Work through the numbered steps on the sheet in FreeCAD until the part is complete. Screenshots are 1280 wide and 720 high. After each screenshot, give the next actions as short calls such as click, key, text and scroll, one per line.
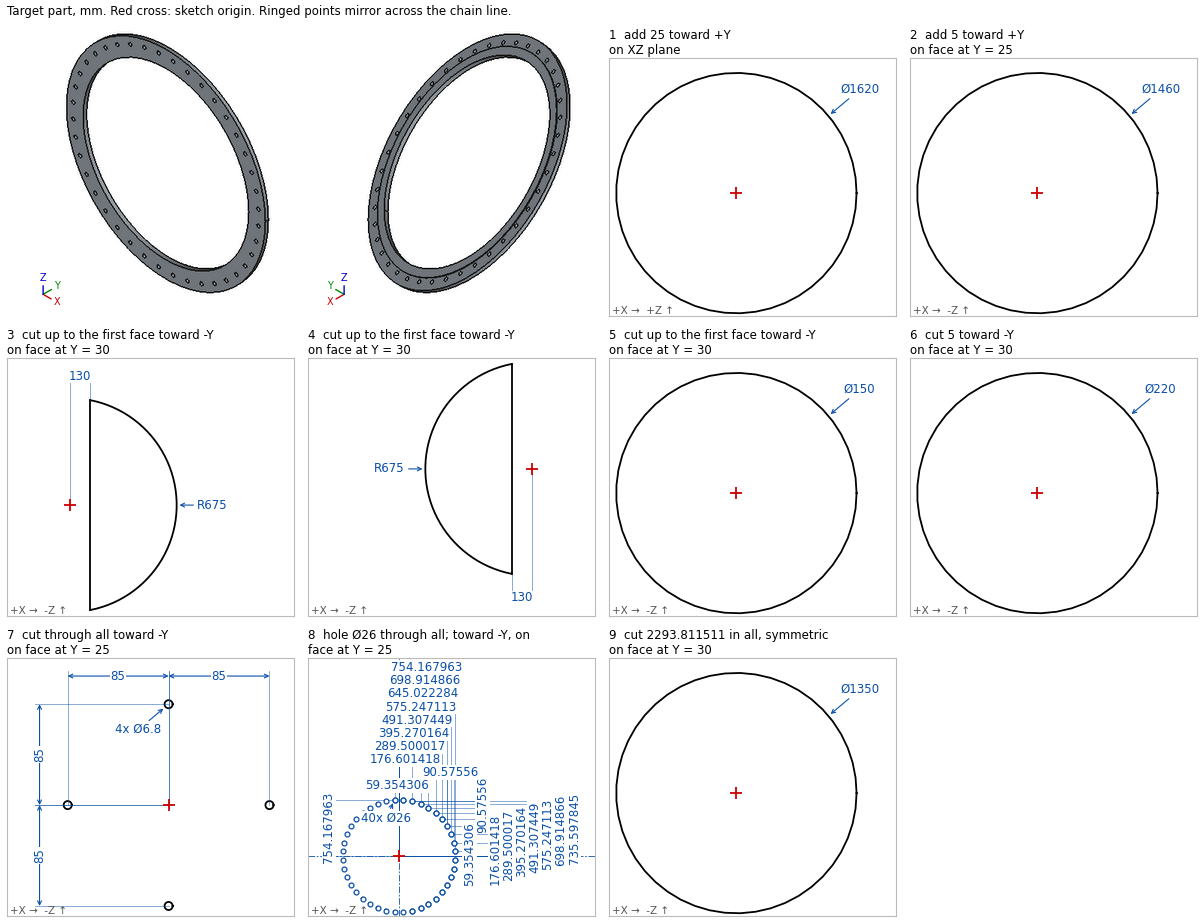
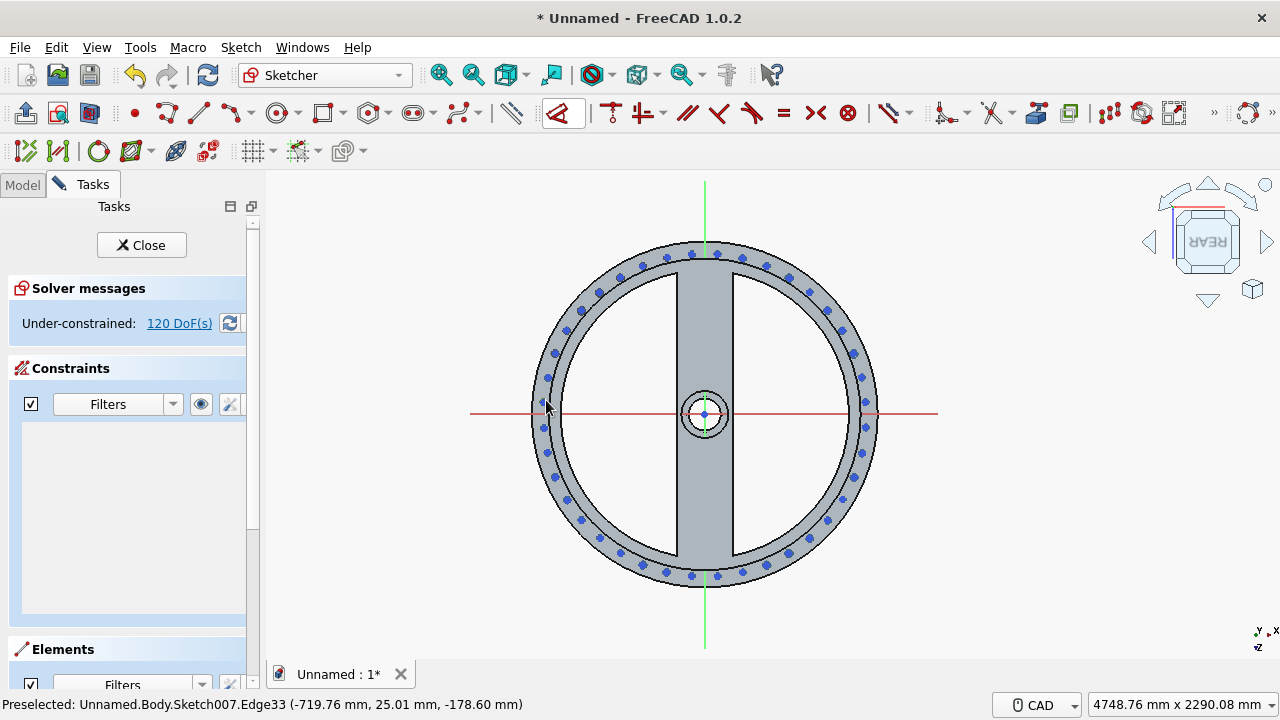
scroll(558, 351, up, 7)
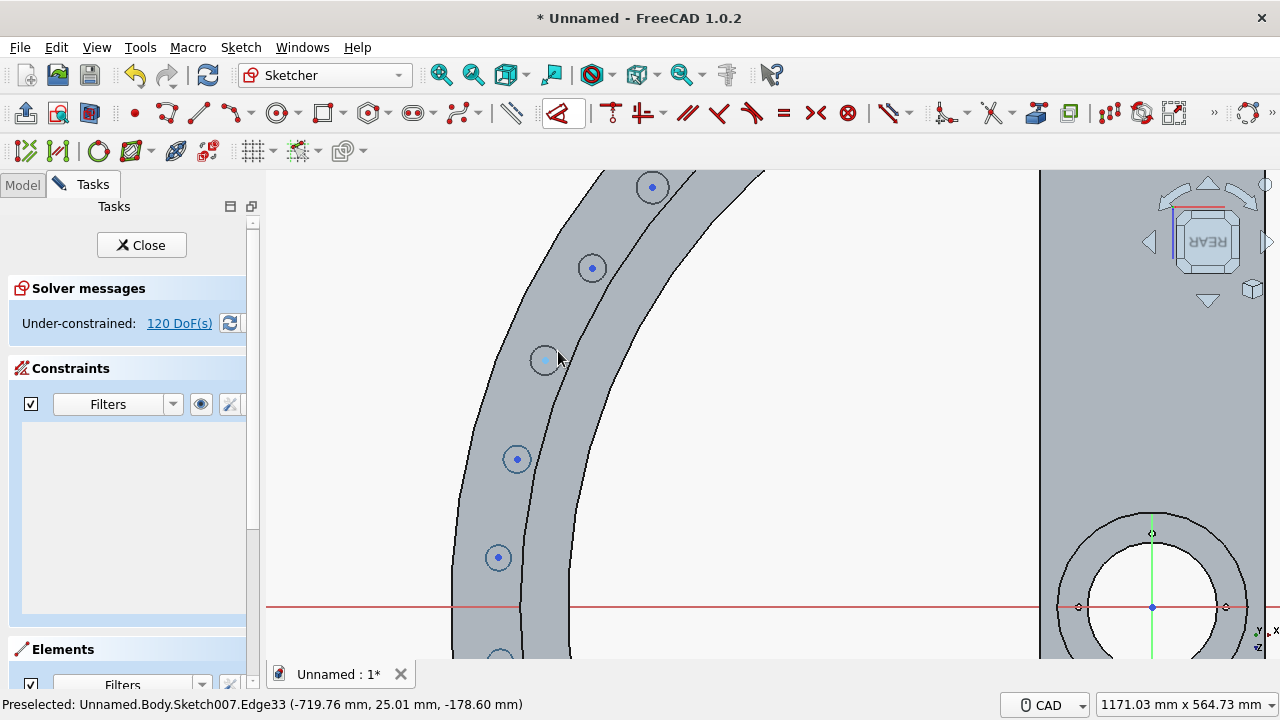
click(555, 350)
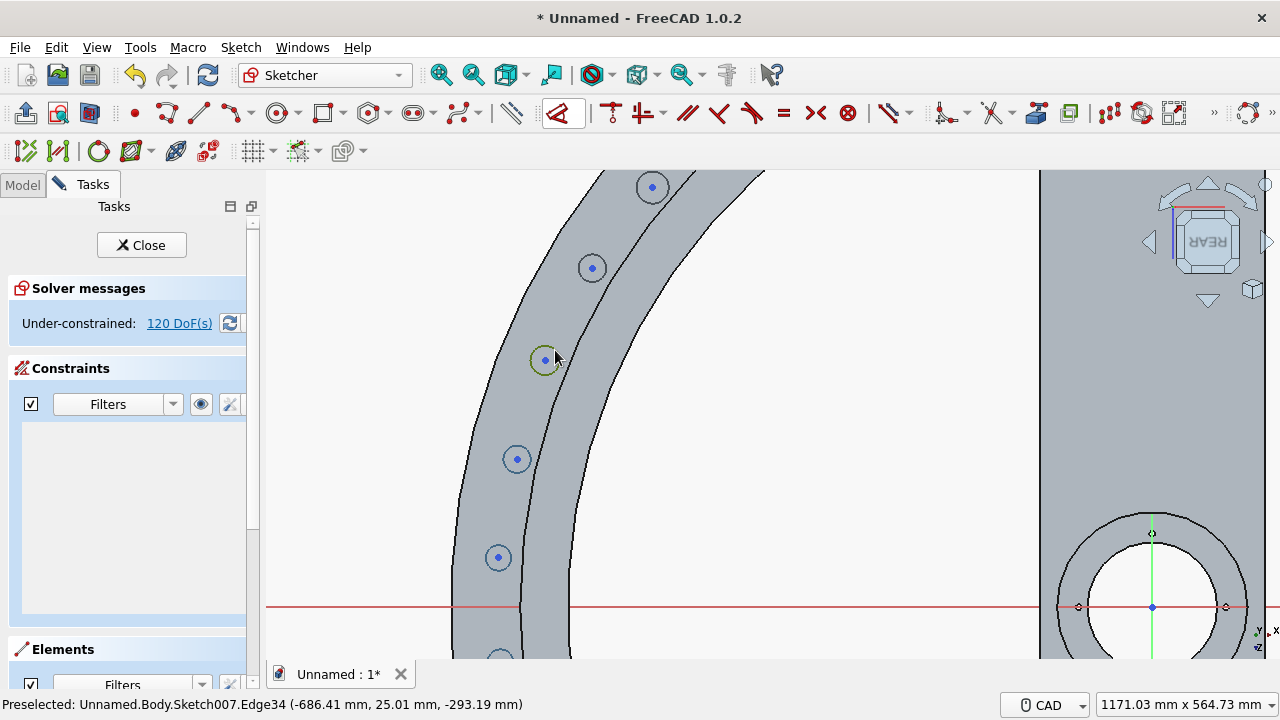
click(602, 258)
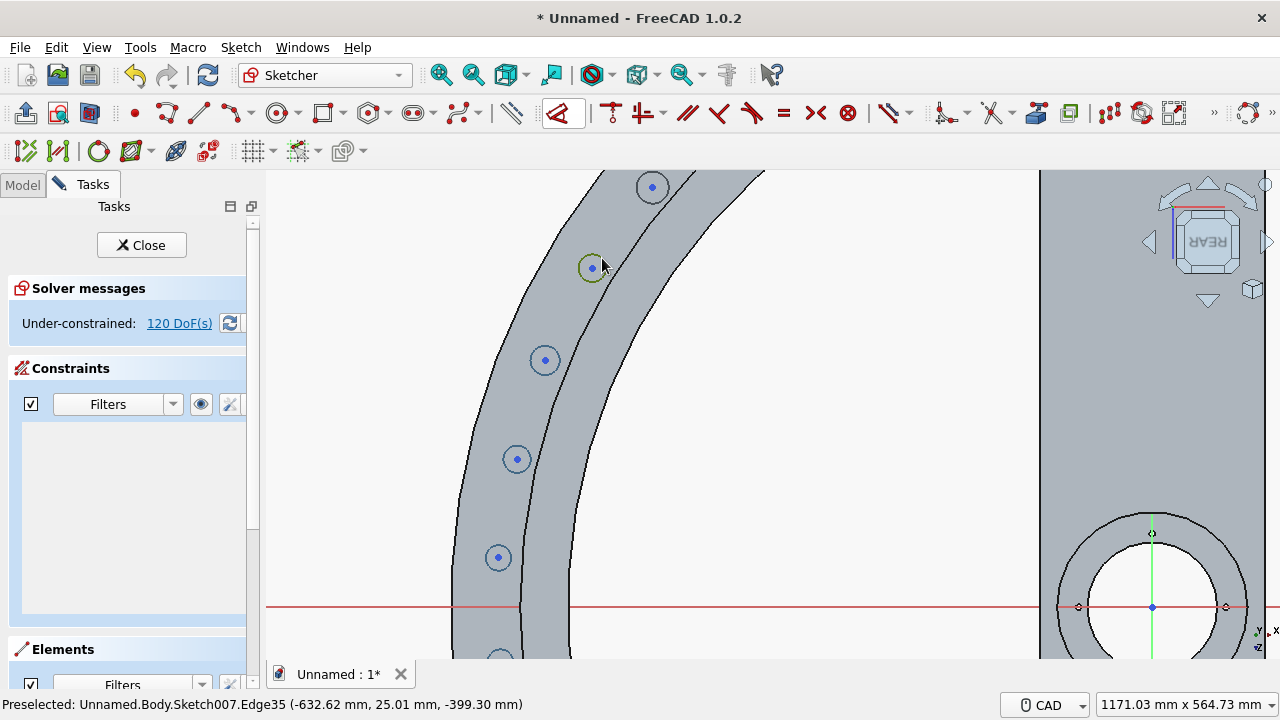
click(641, 199)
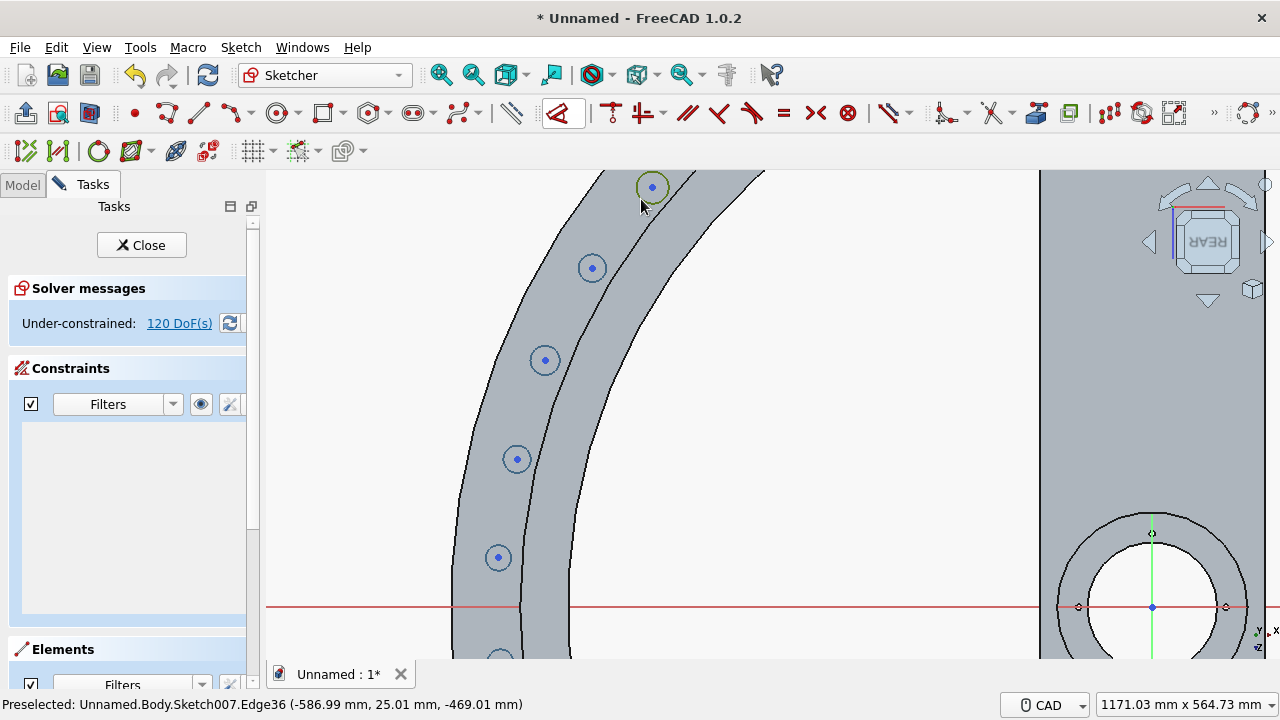
scroll(558, 351, down, 7)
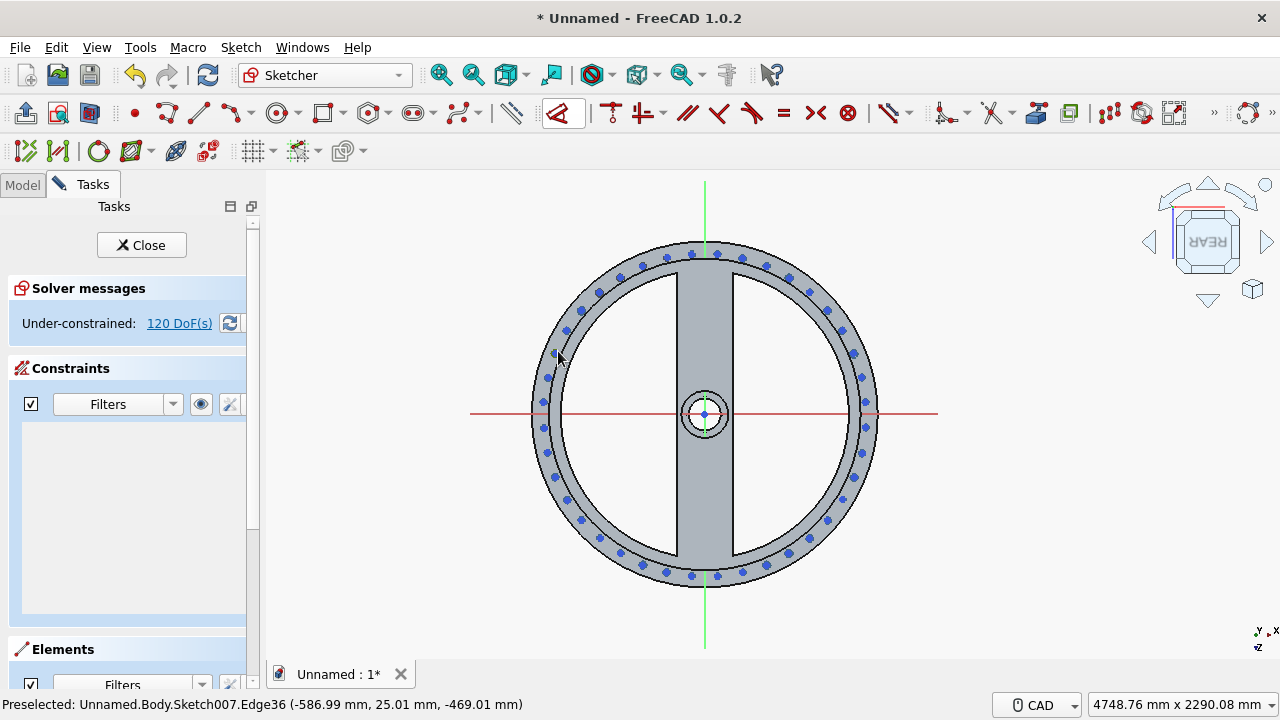
scroll(602, 290, up, 7)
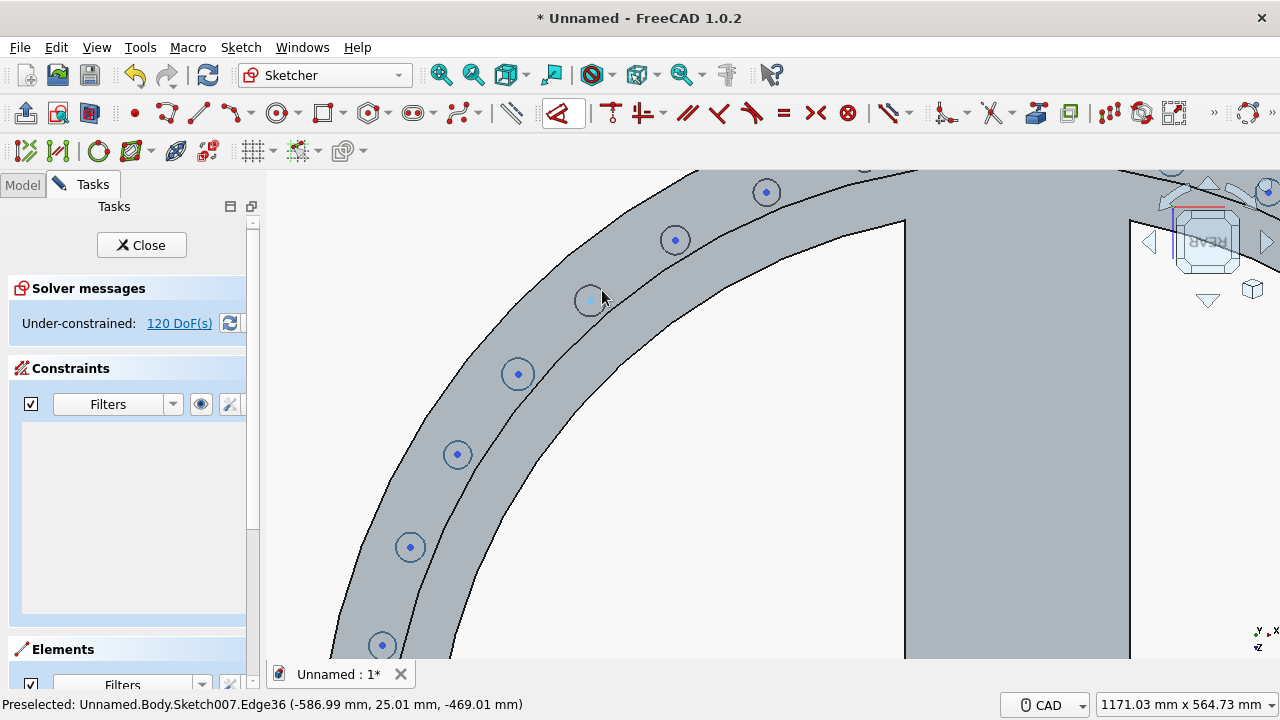
click(601, 290)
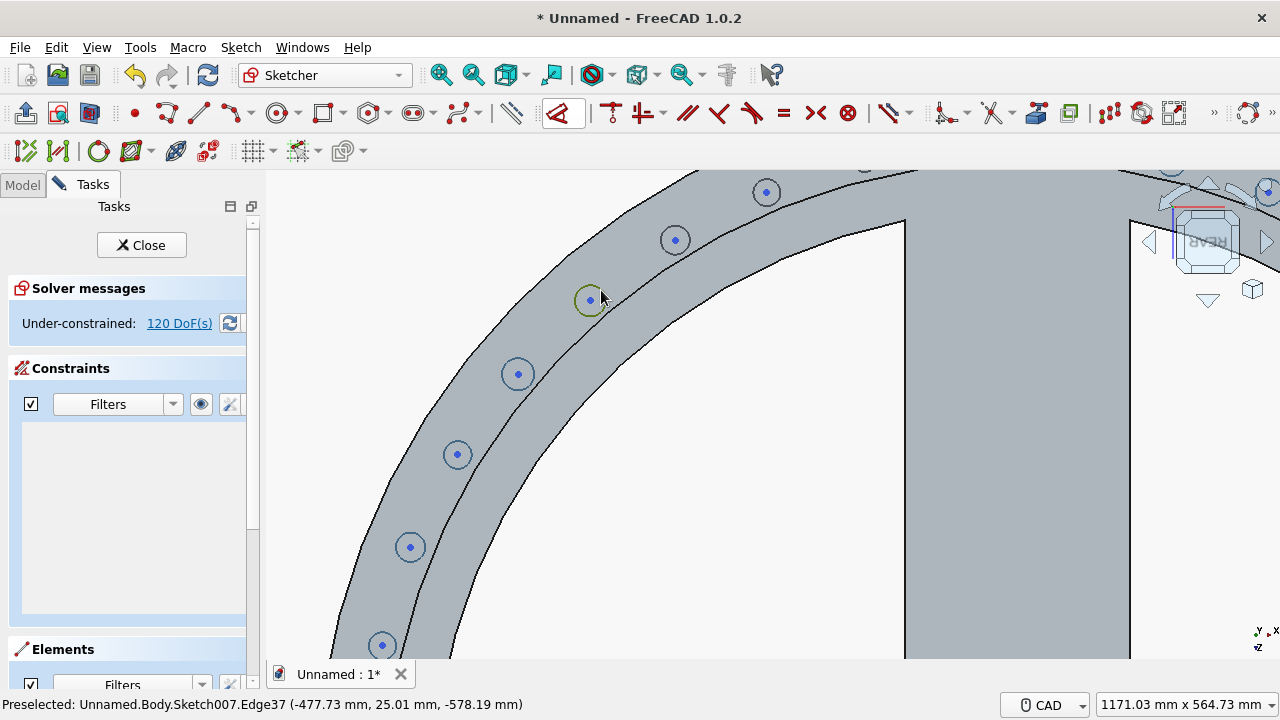
click(686, 230)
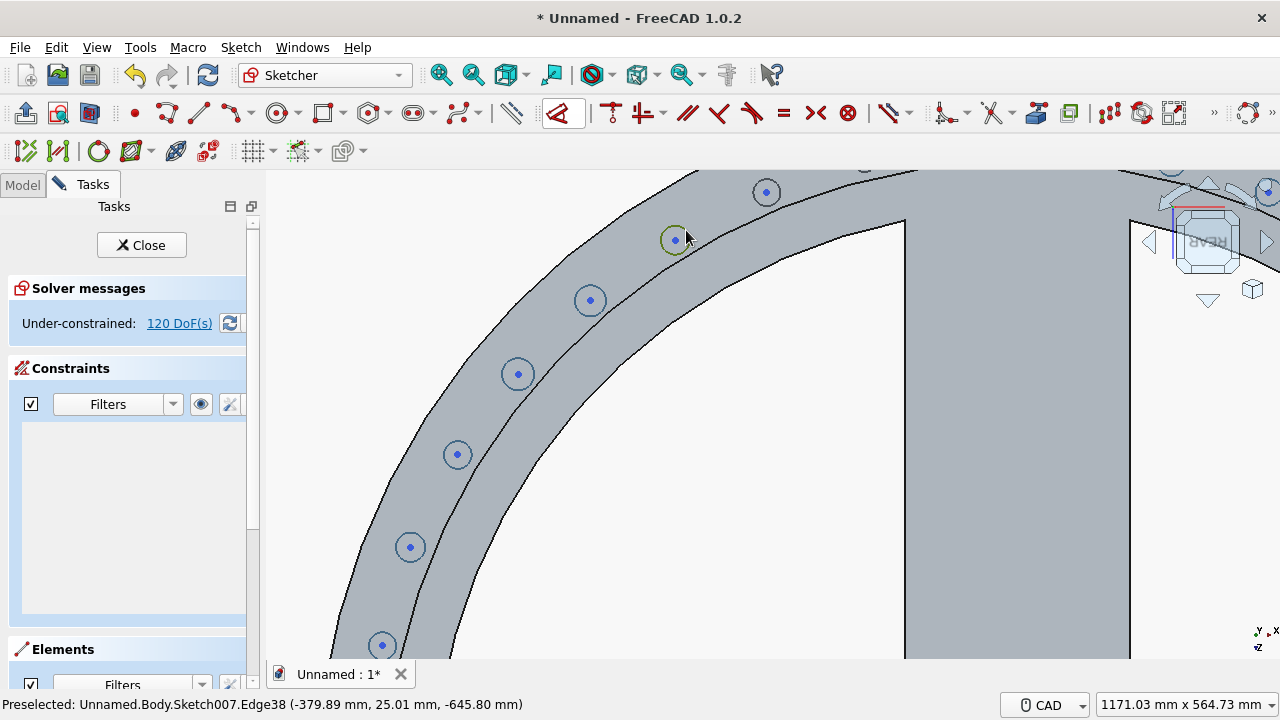
click(757, 202)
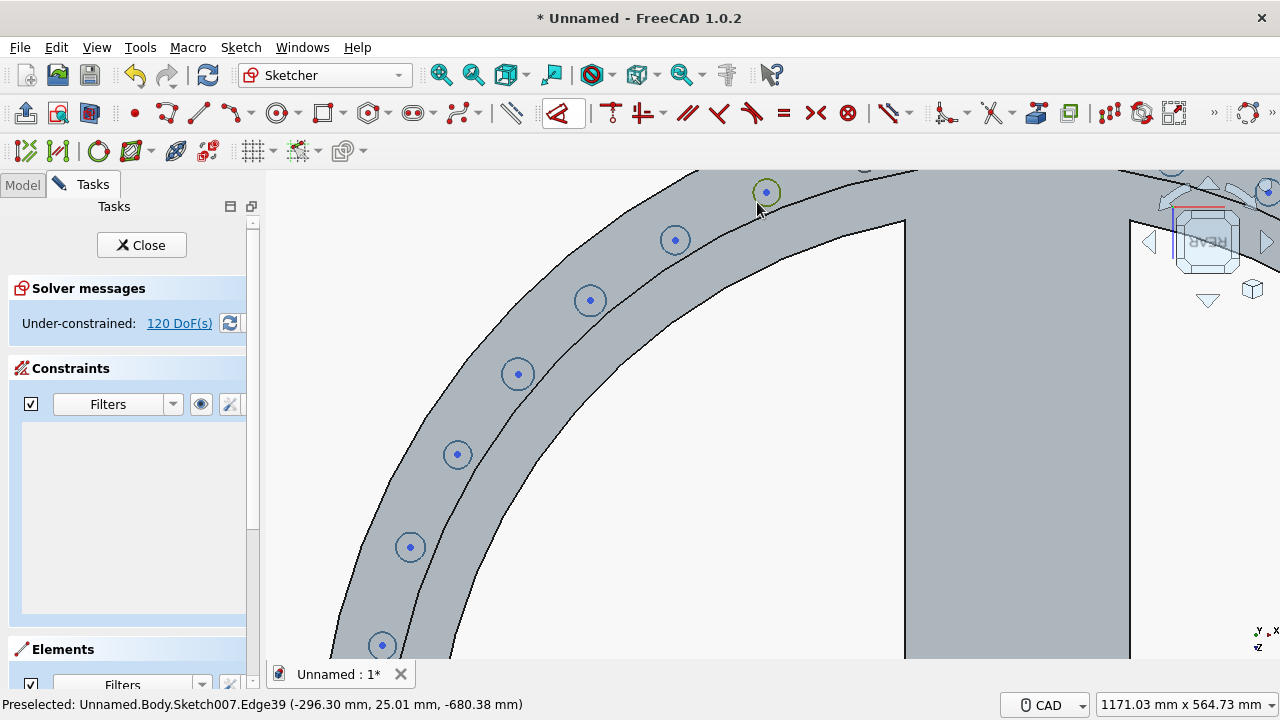
scroll(602, 290, down, 7)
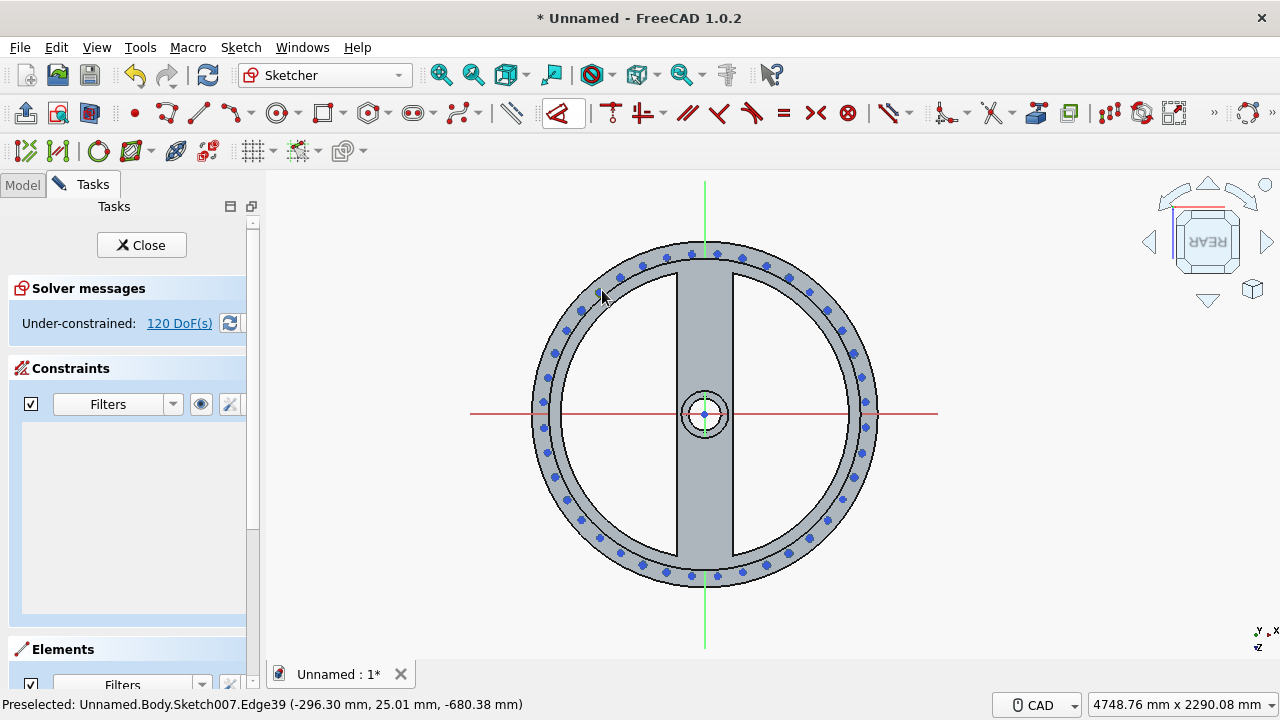
scroll(669, 256, up, 8)